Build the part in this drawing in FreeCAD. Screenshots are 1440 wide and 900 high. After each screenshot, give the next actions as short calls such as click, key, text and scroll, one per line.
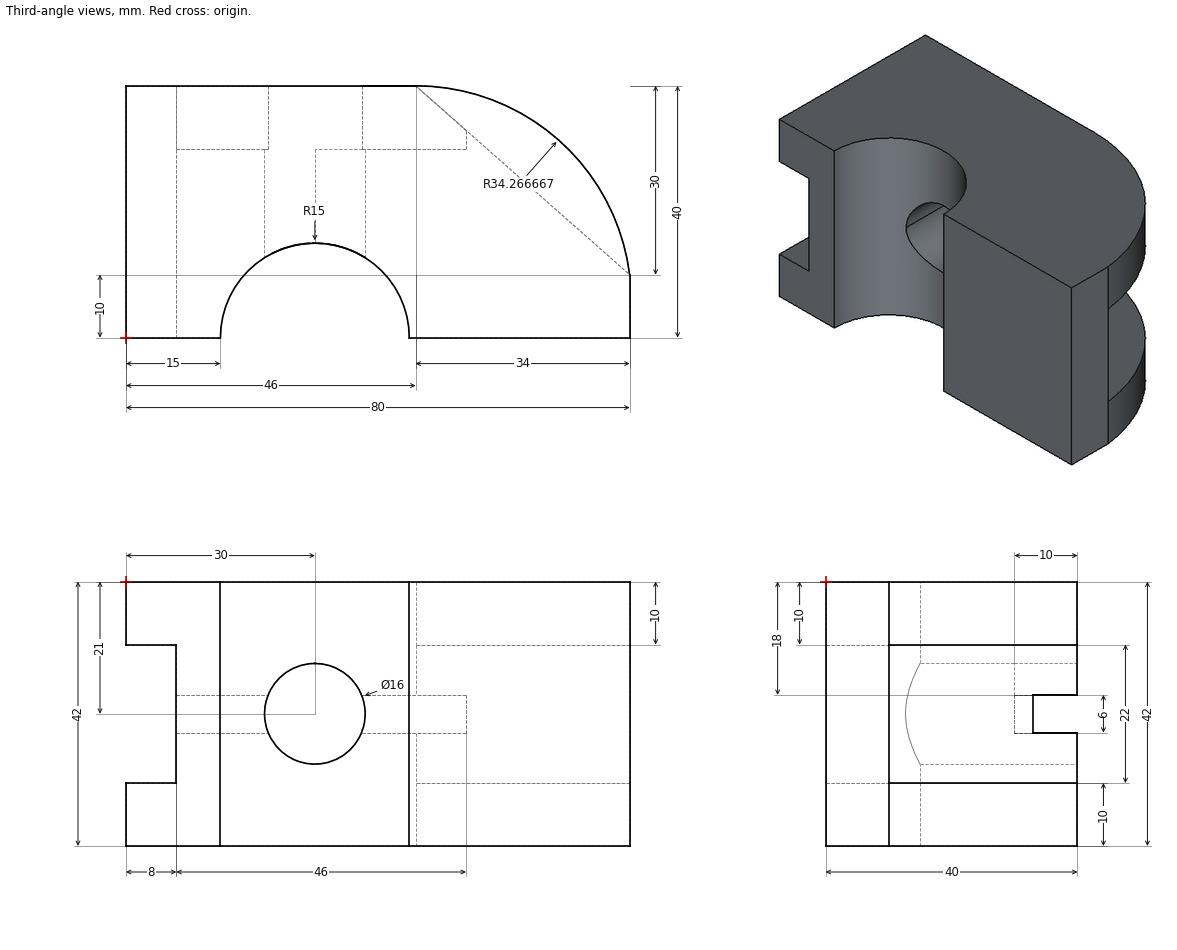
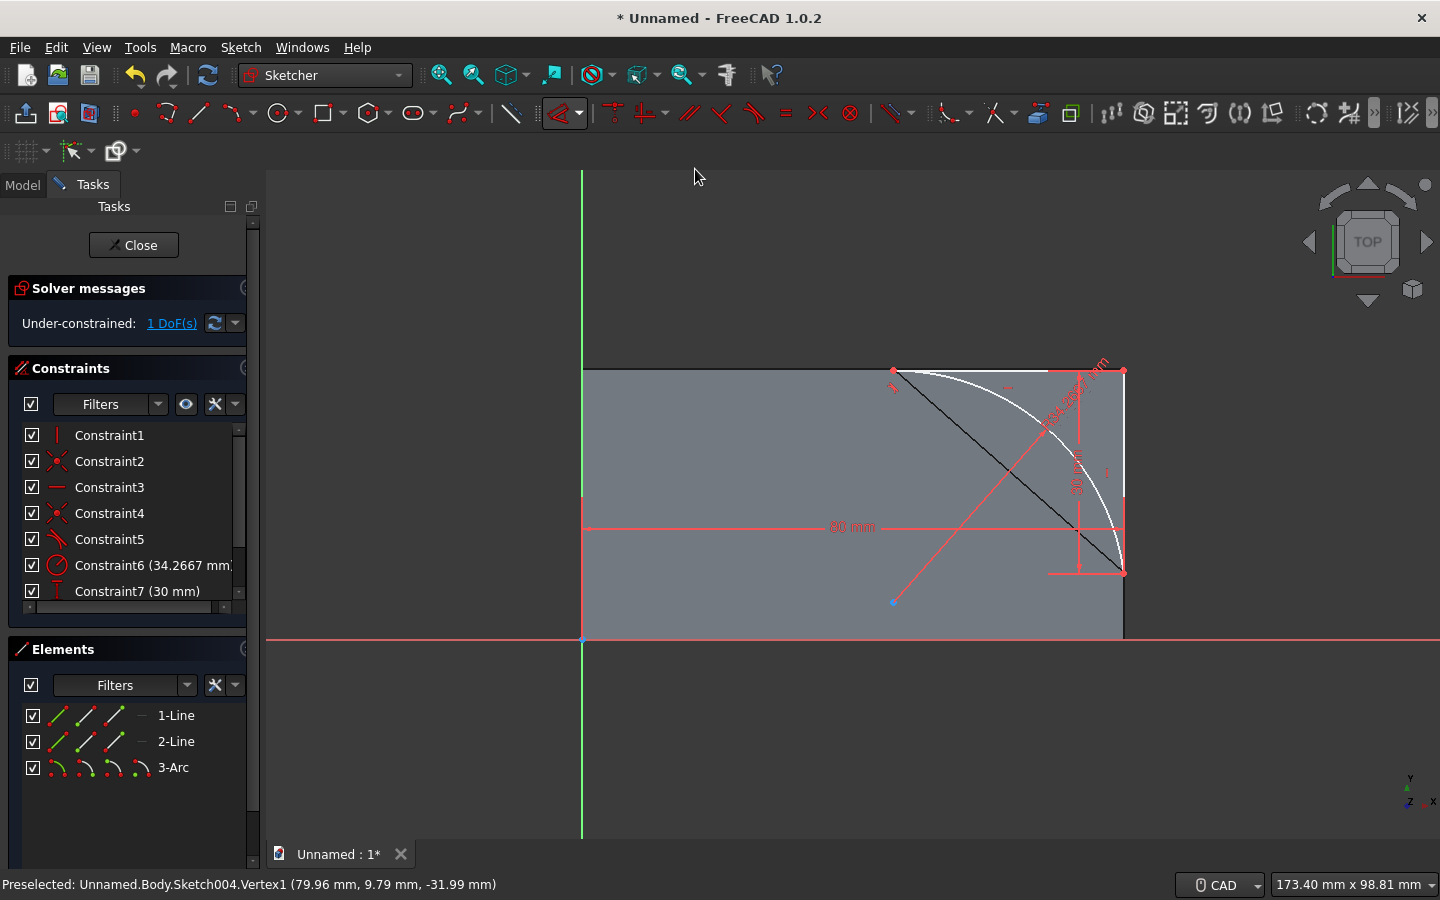
click(1124, 574)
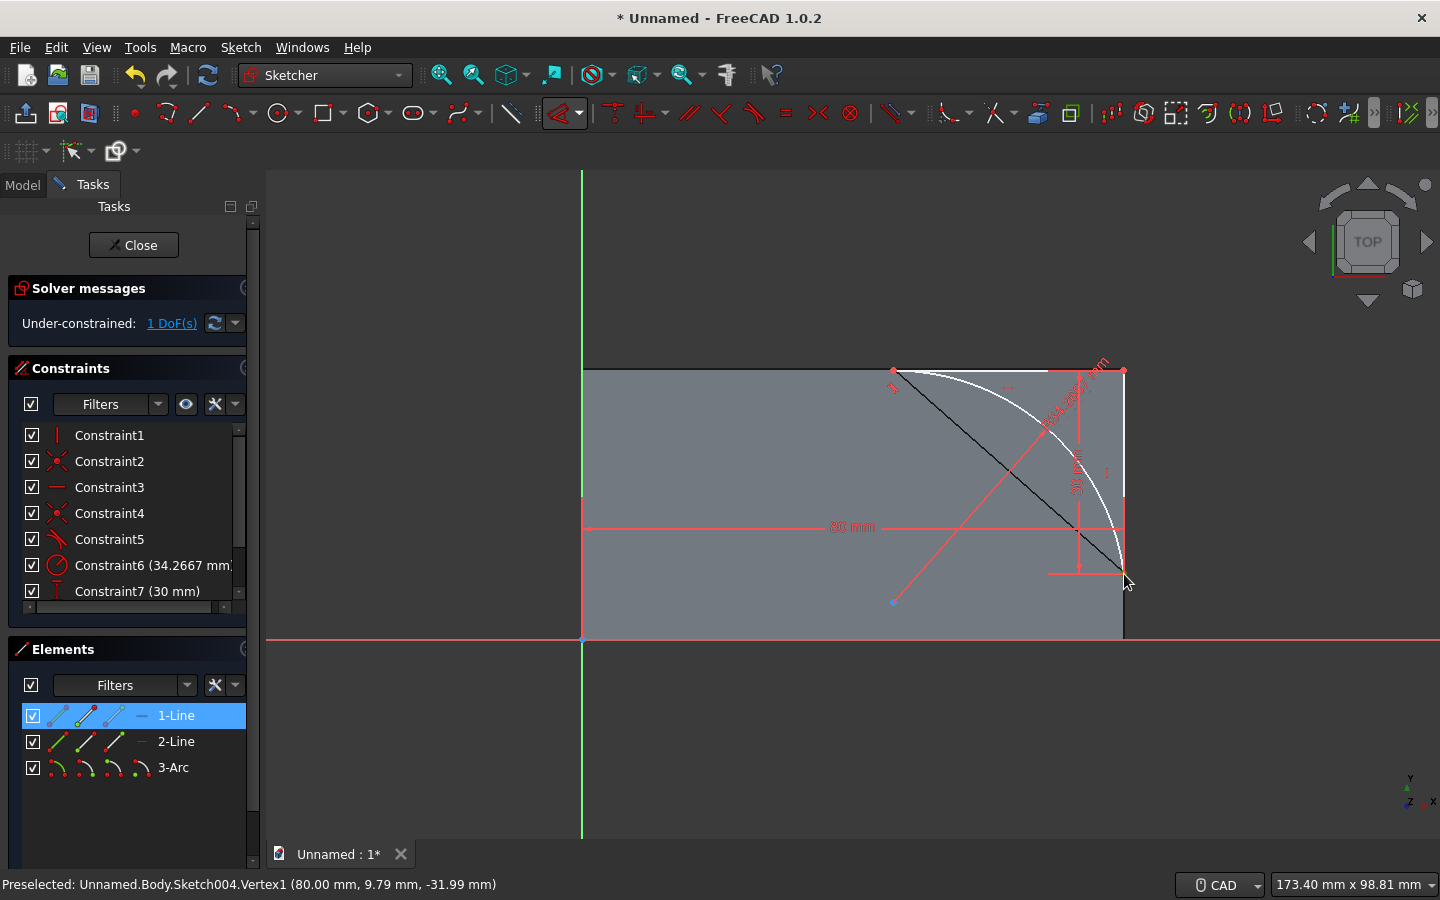
key(i)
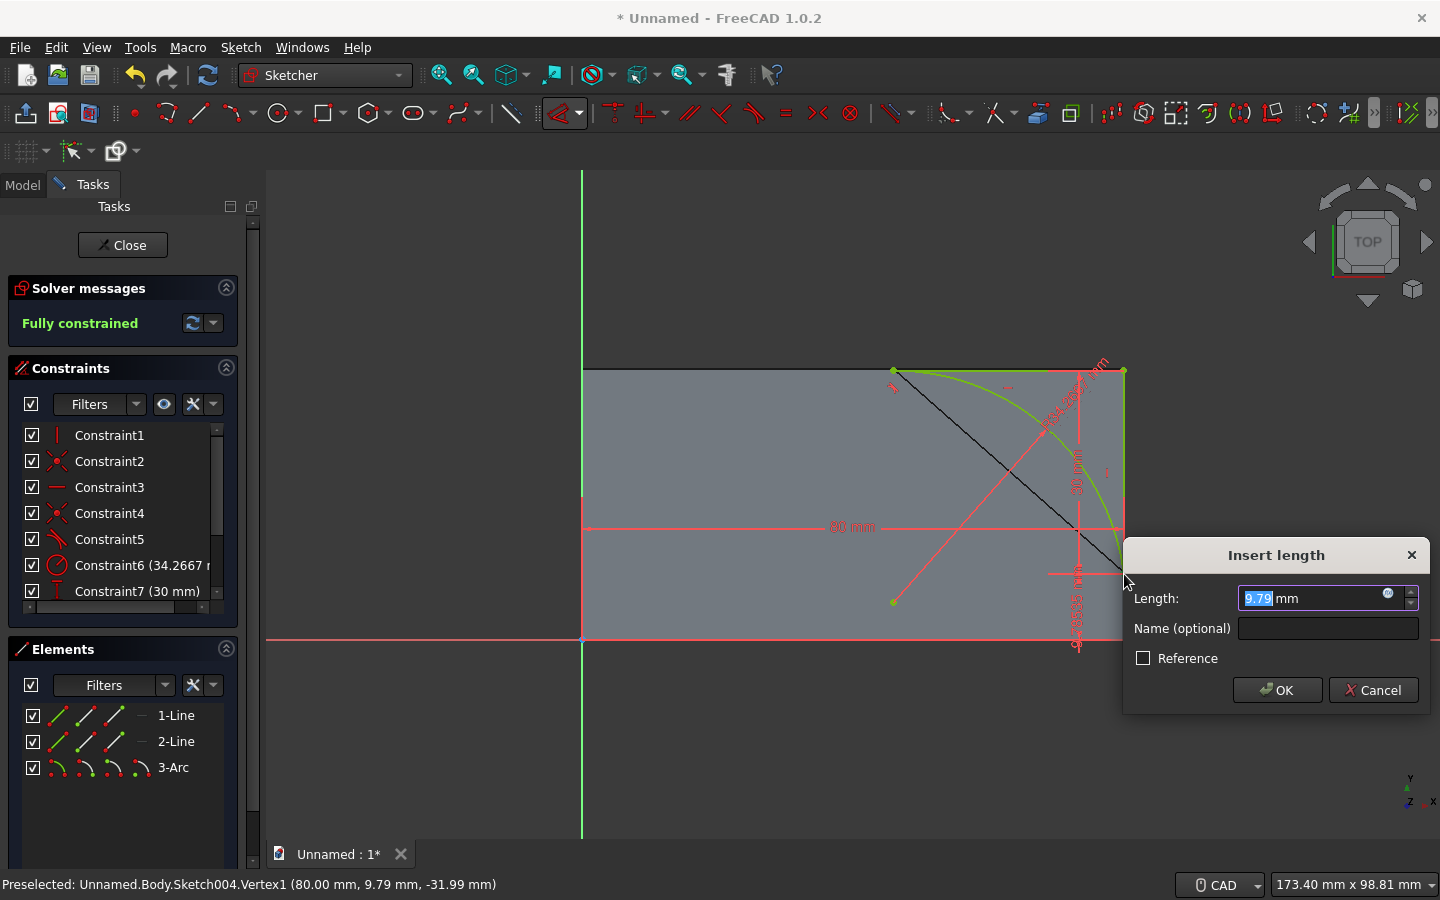
text(10)
key(Return)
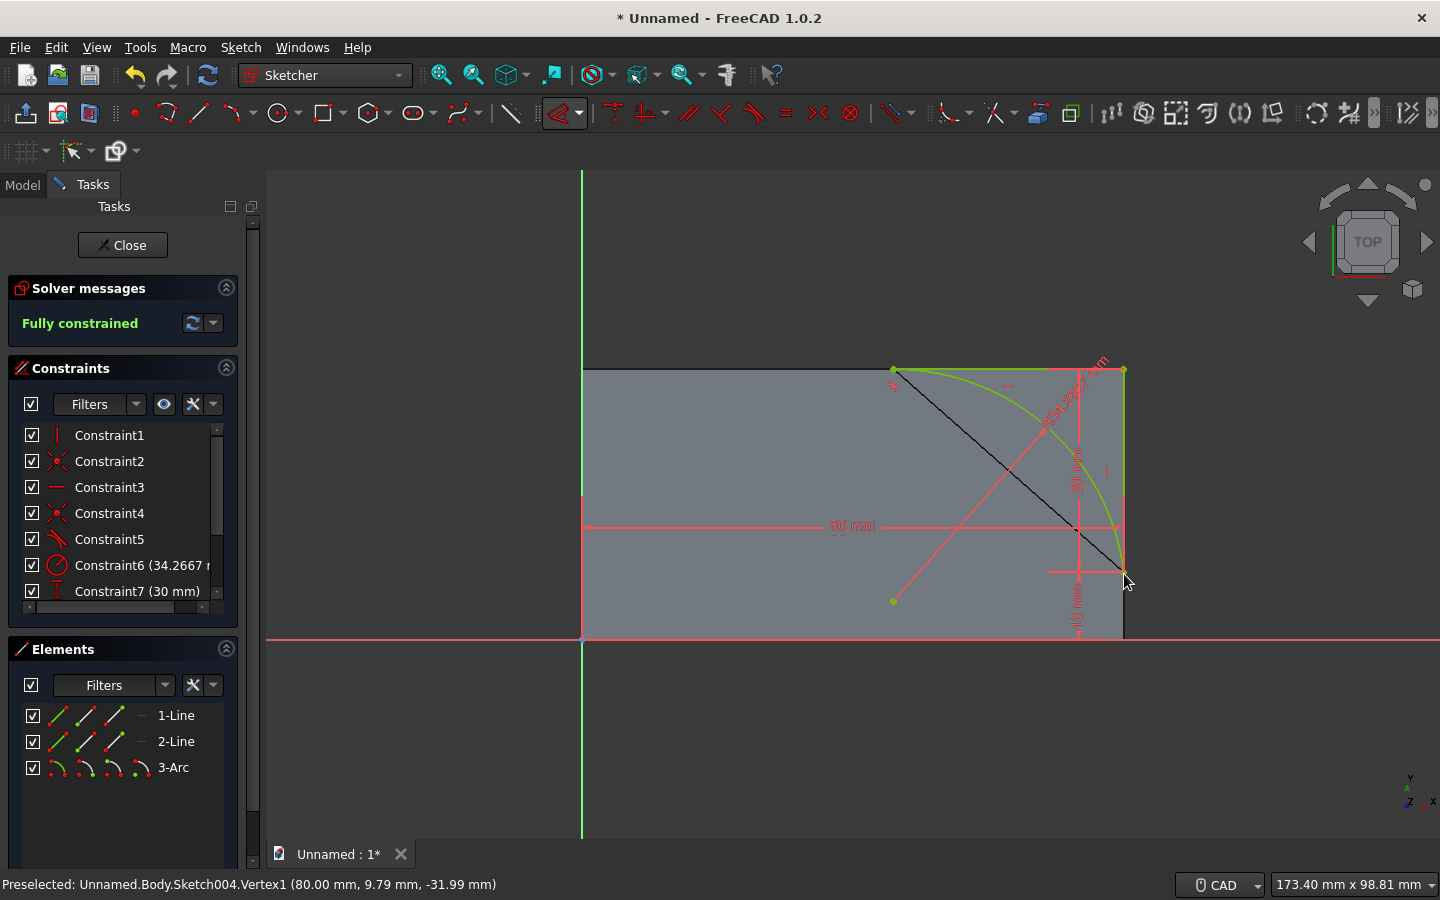
click(123, 245)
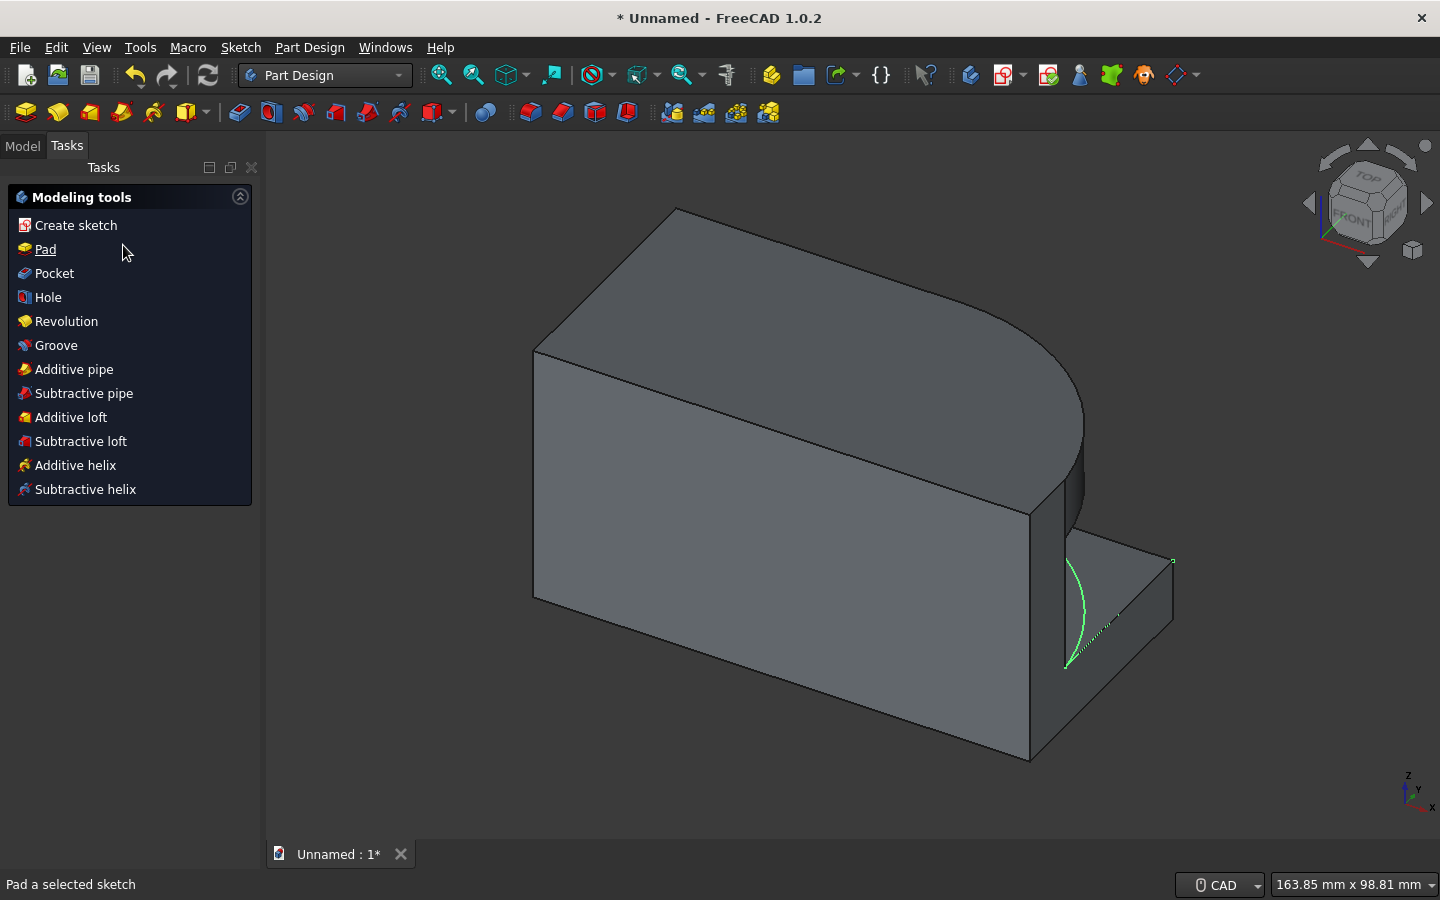
click(240, 112)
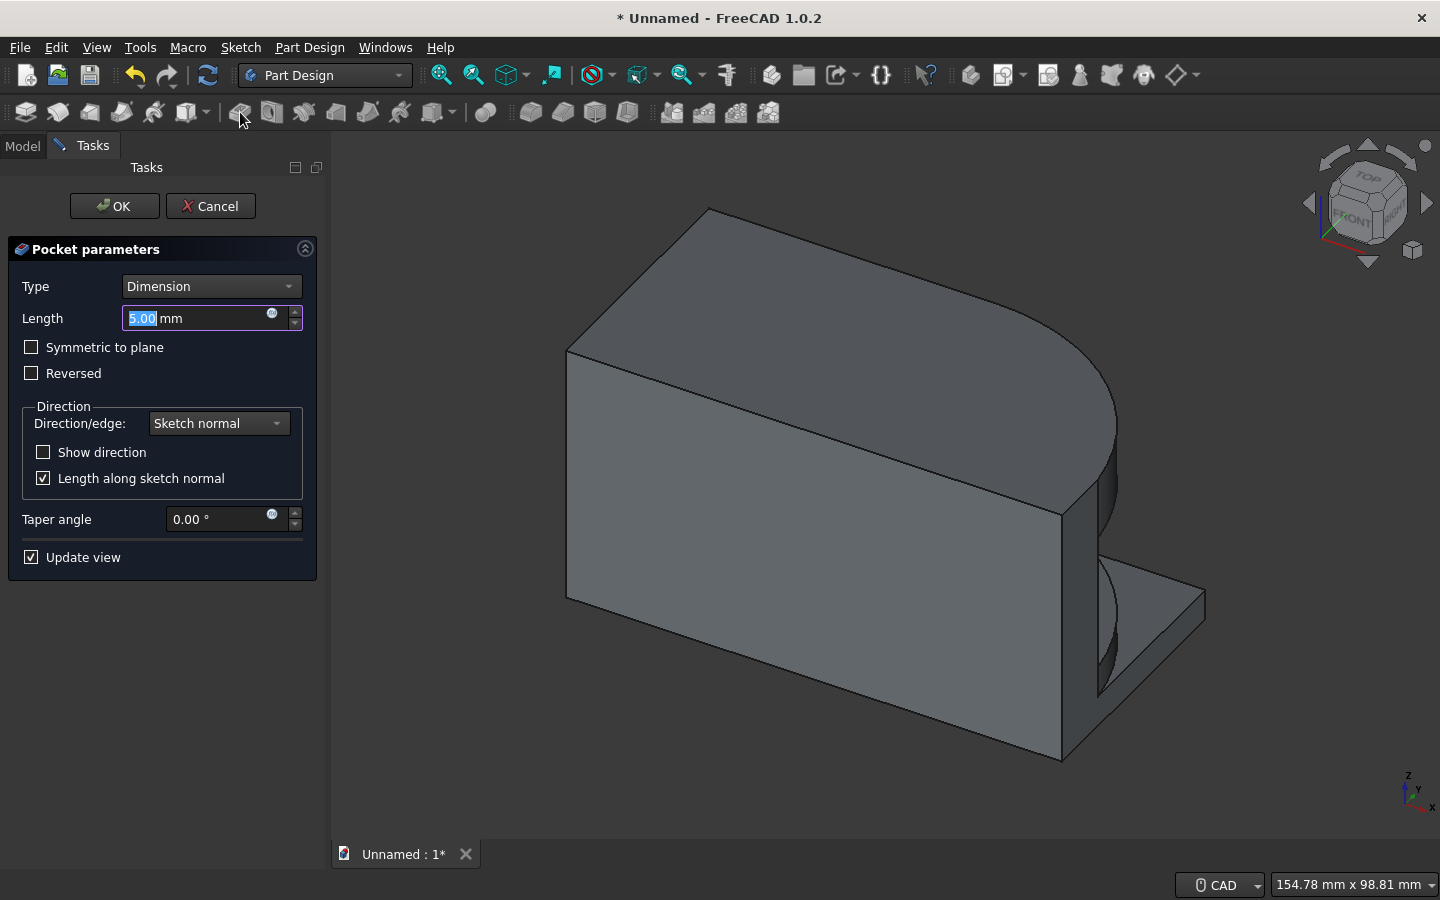
text(10)
key(Tab)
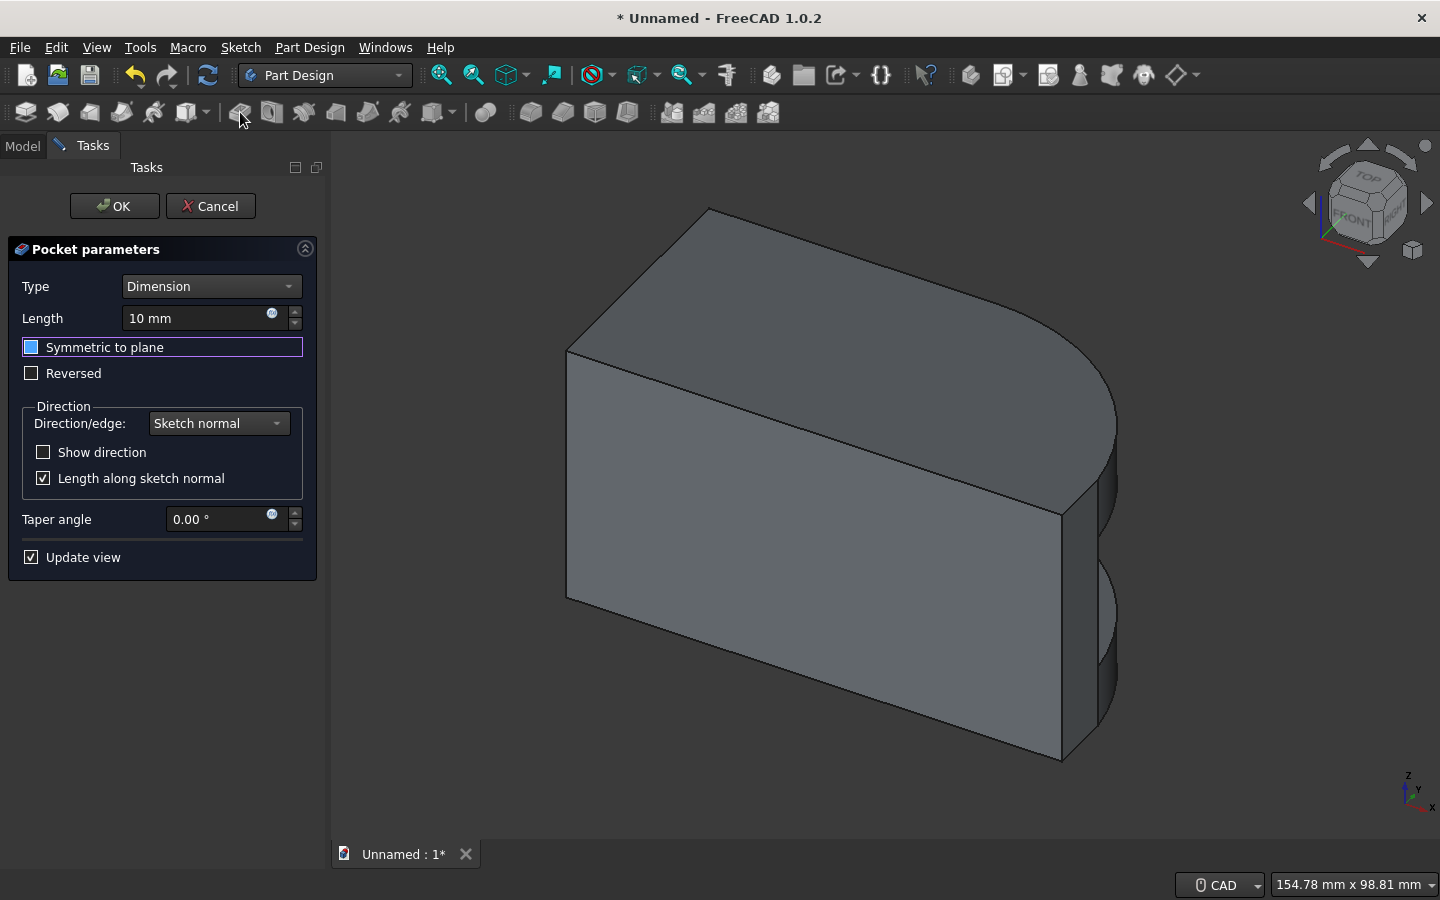
click(115, 206)